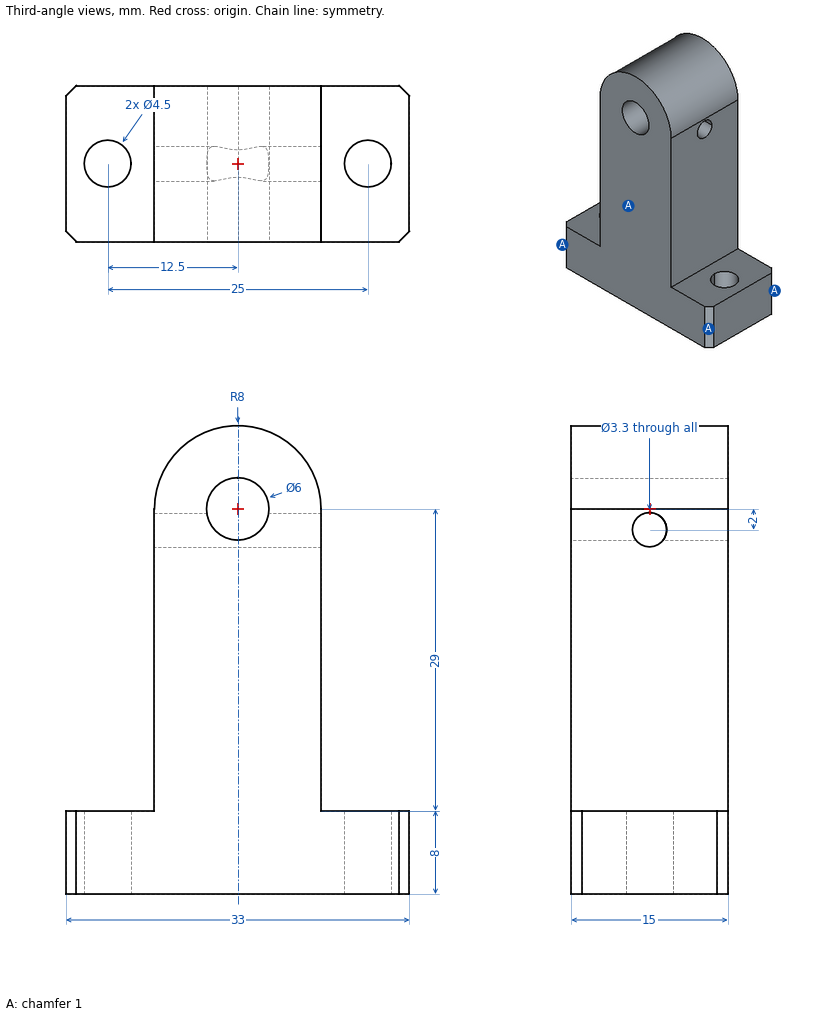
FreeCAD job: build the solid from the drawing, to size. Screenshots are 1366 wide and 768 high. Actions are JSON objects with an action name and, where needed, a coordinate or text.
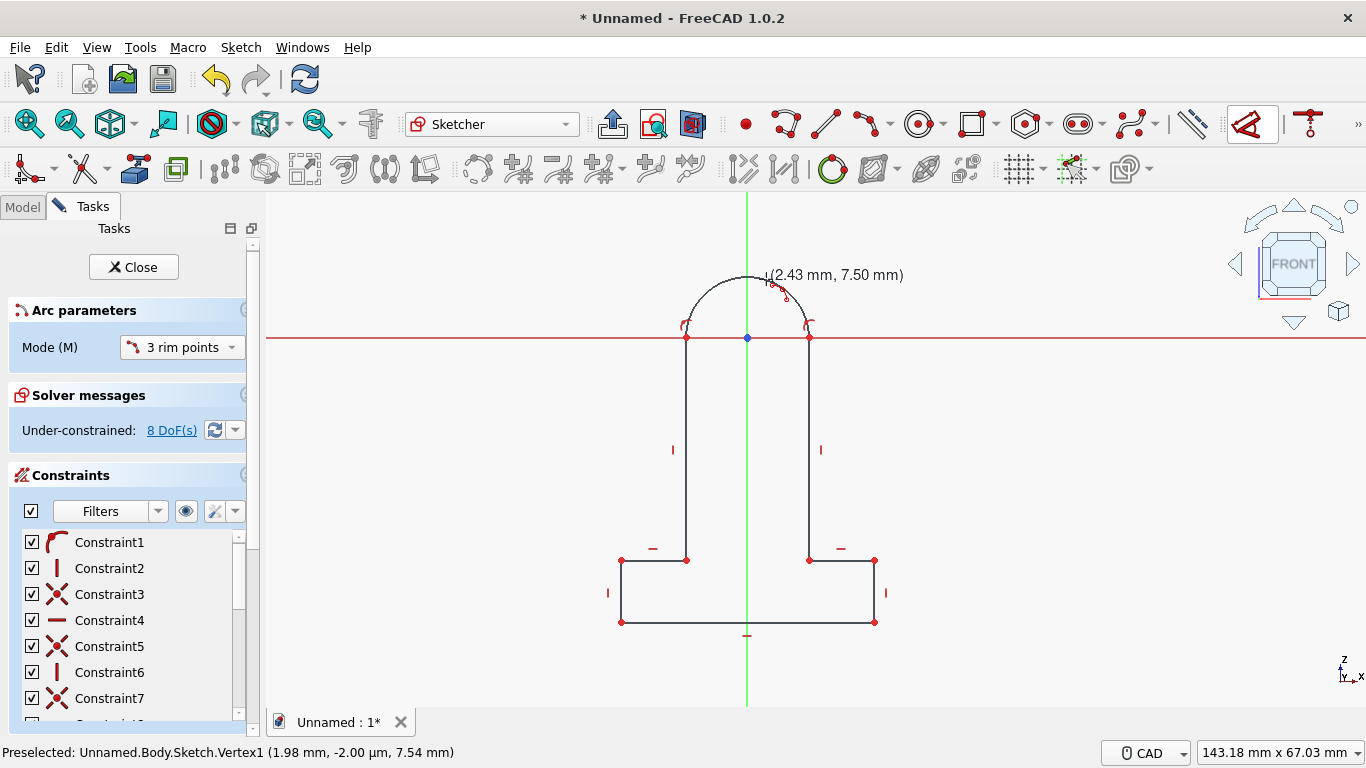
{"action": "left_click", "coordinate": [920, 124]}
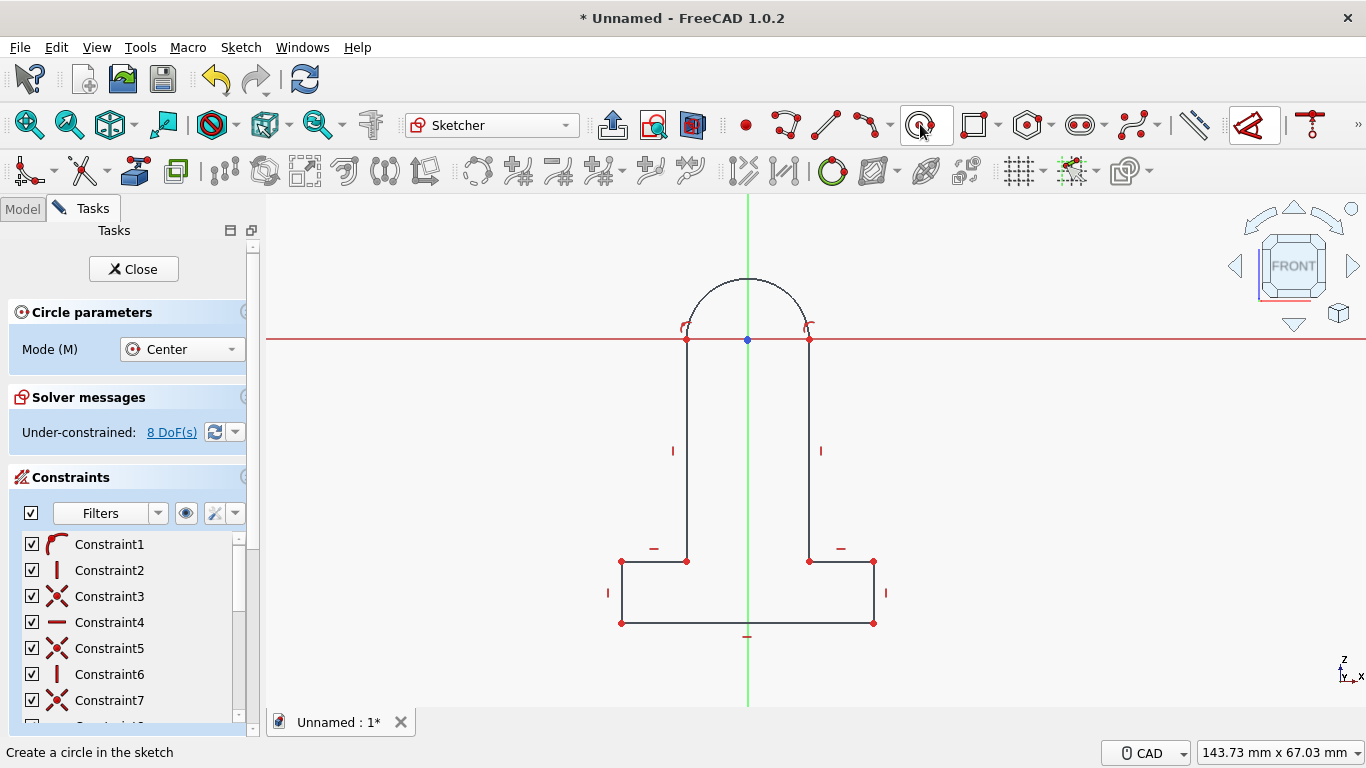
{"action": "left_click", "coordinate": [748, 339]}
{"action": "mouse_move", "coordinate": [764, 323]}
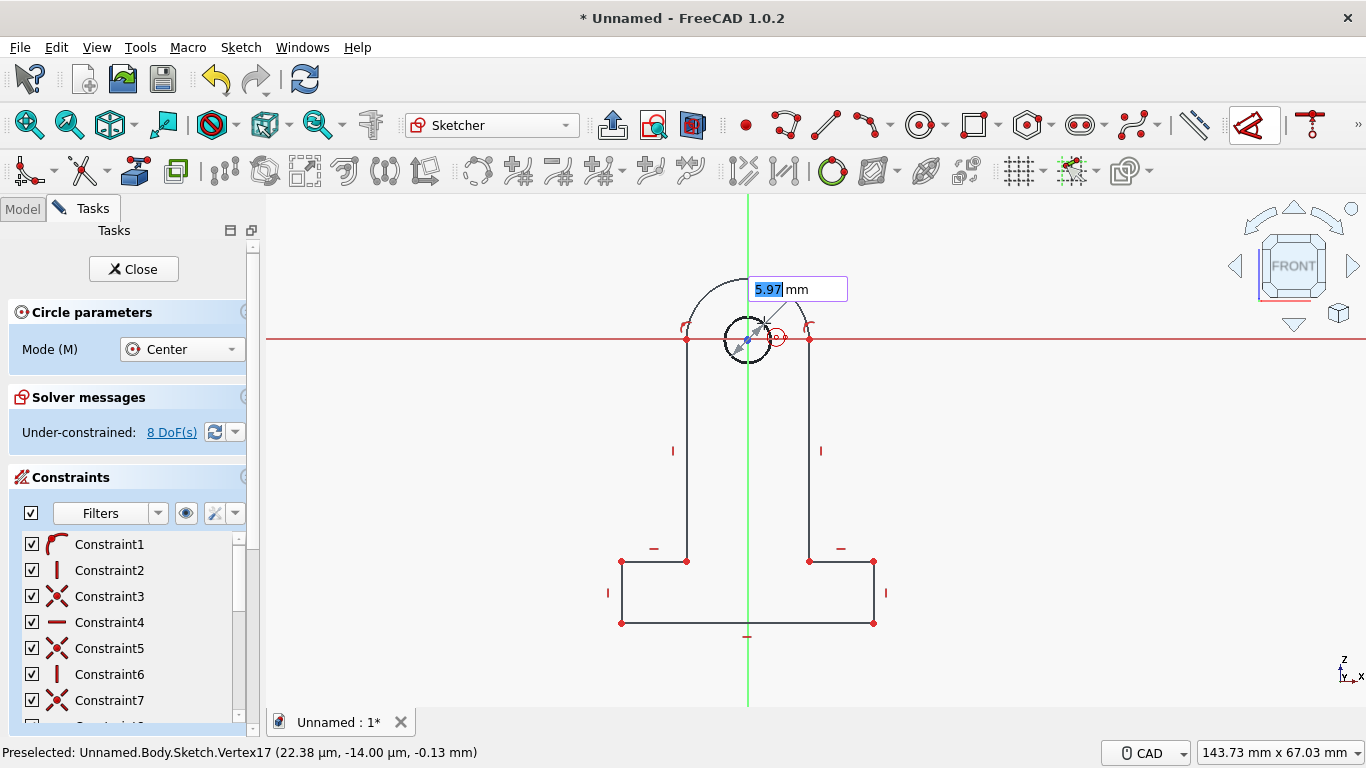
{"action": "type", "text": "6"}
{"action": "key", "text": "Return"}
{"action": "key", "text": "Escape"}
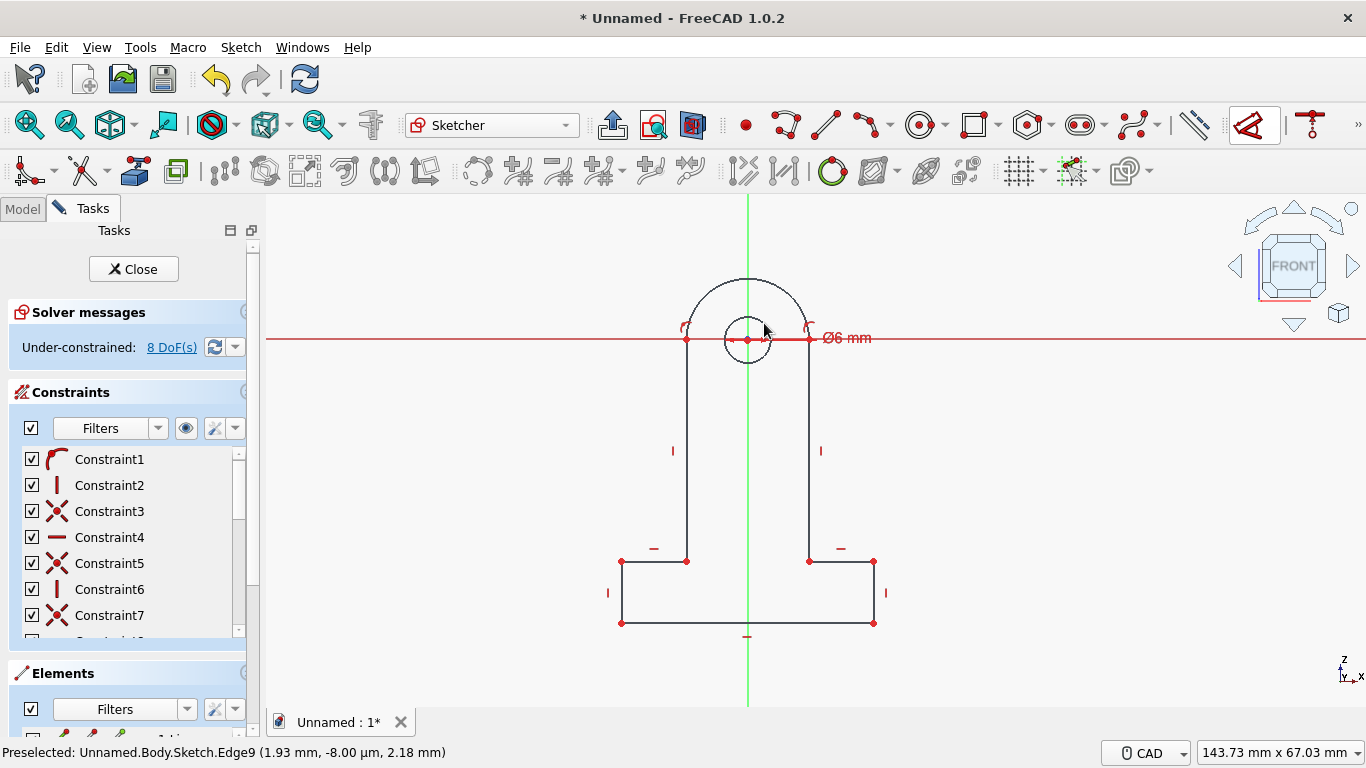
{"action": "left_click", "coordinate": [809, 406]}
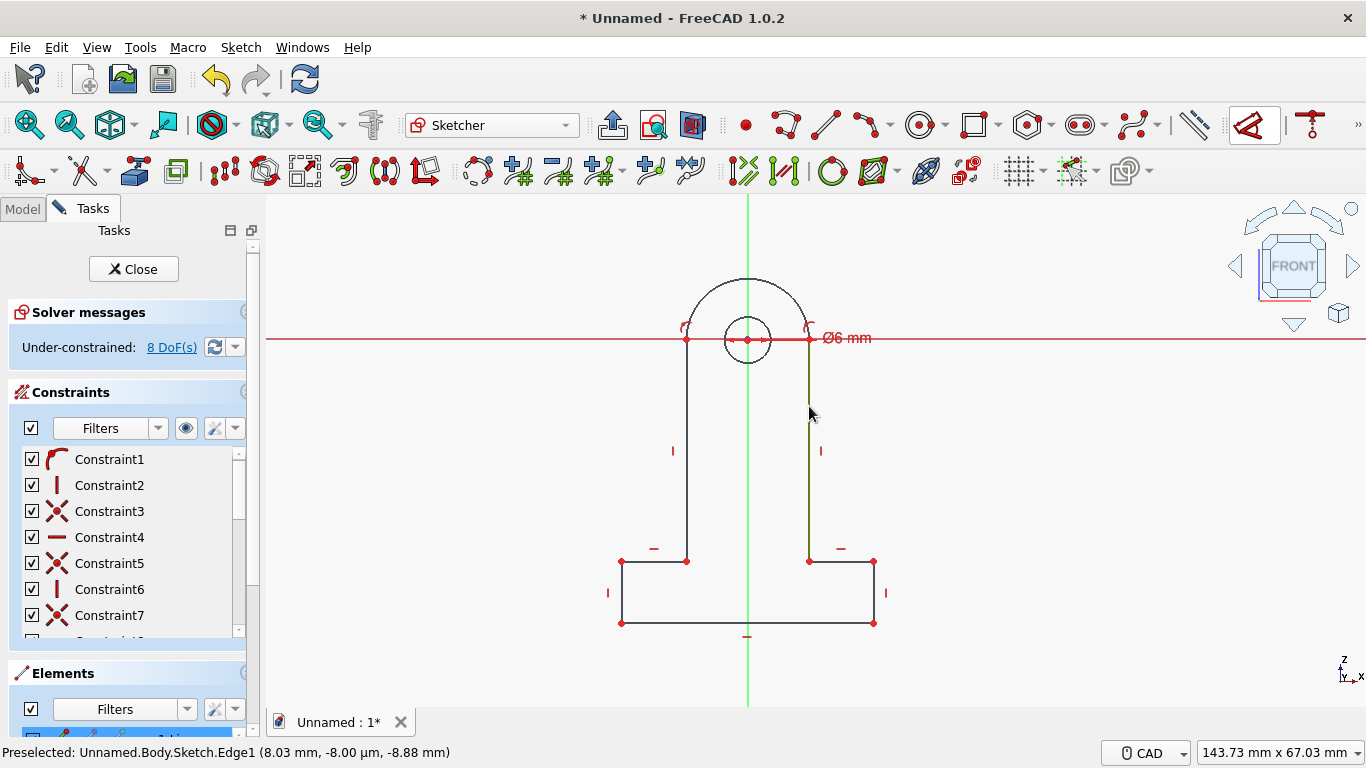
{"action": "left_click", "coordinate": [783, 290]}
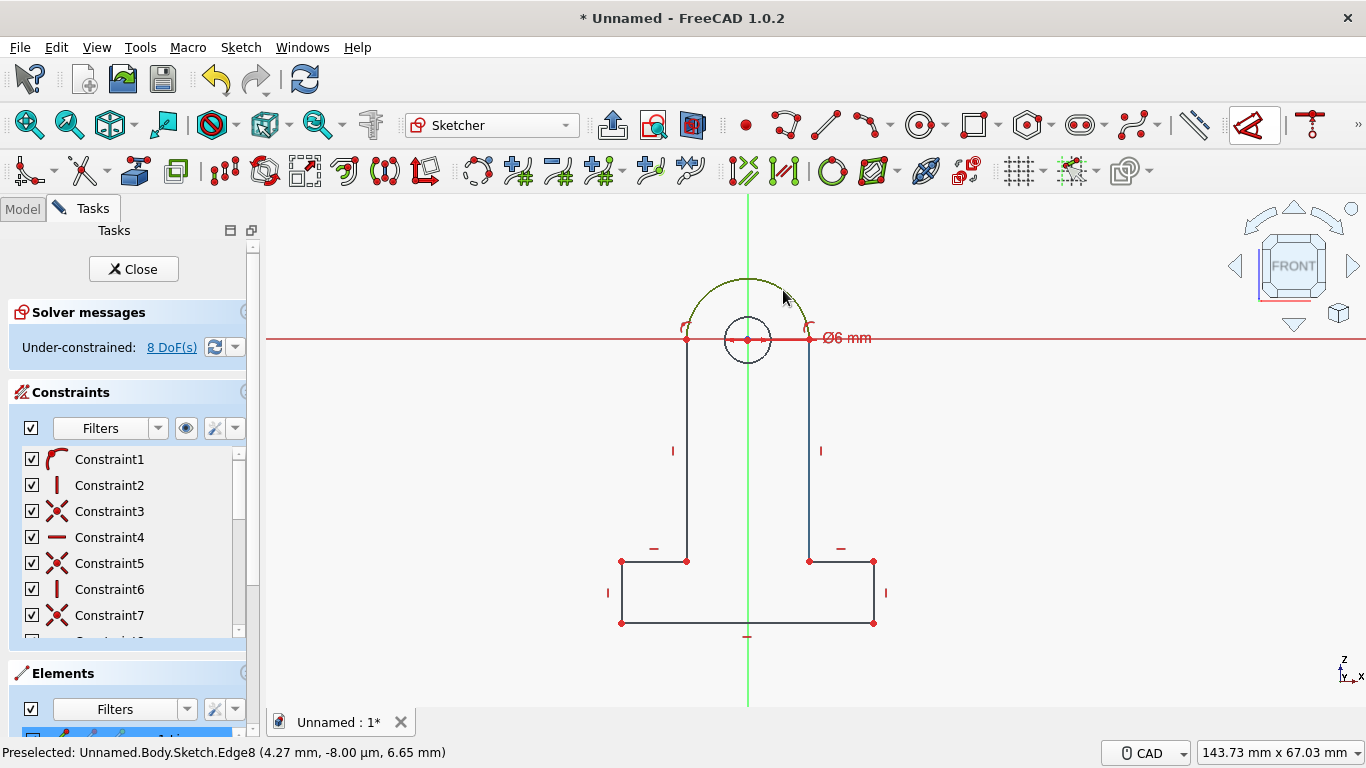
{"action": "key", "text": "t"}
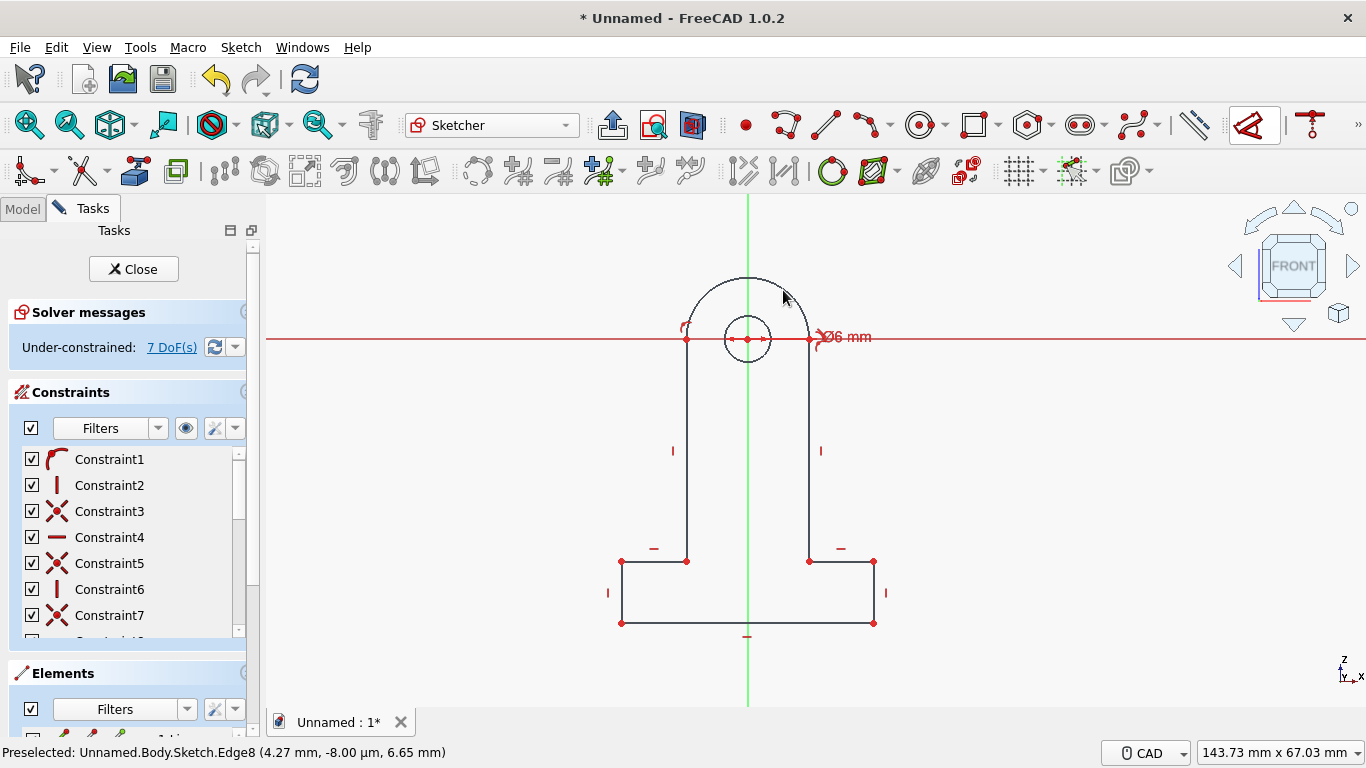
{"action": "left_click", "coordinate": [748, 339]}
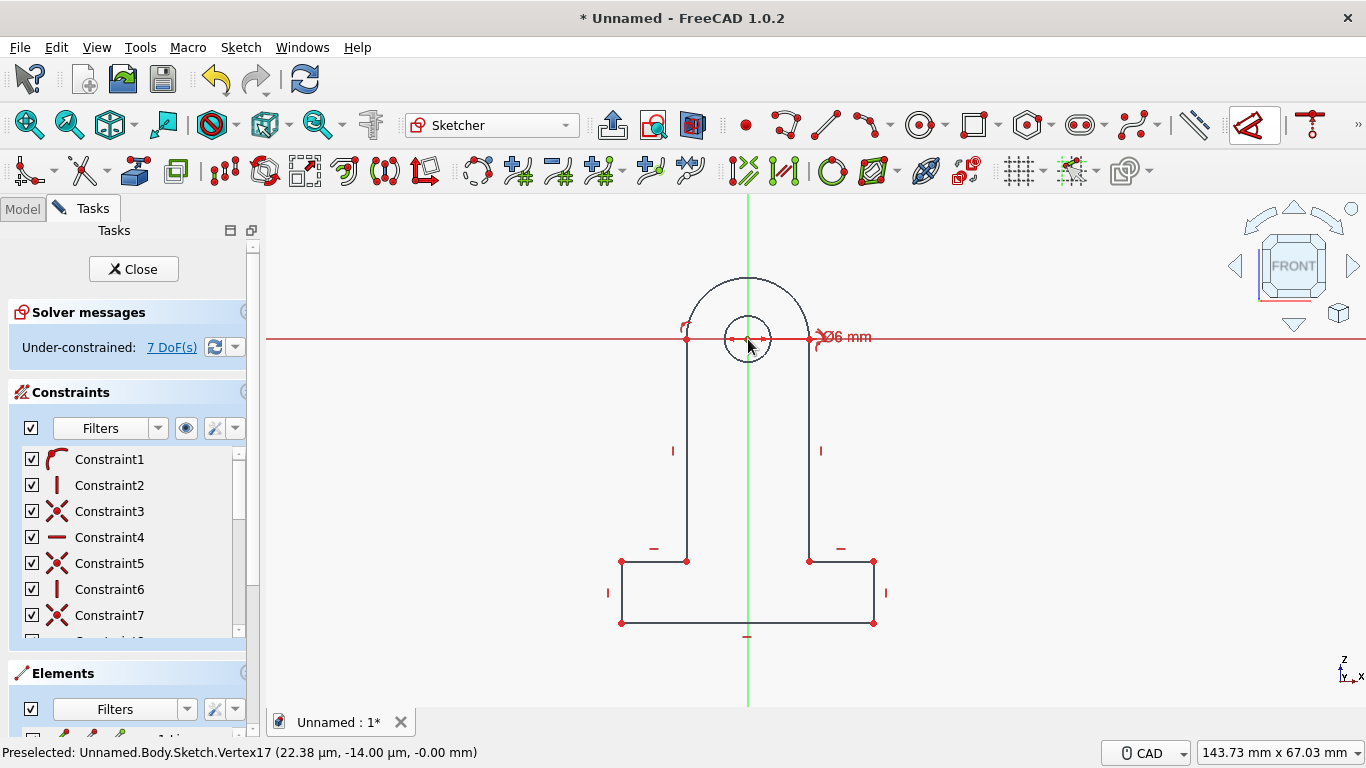
{"action": "left_click", "coordinate": [748, 581]}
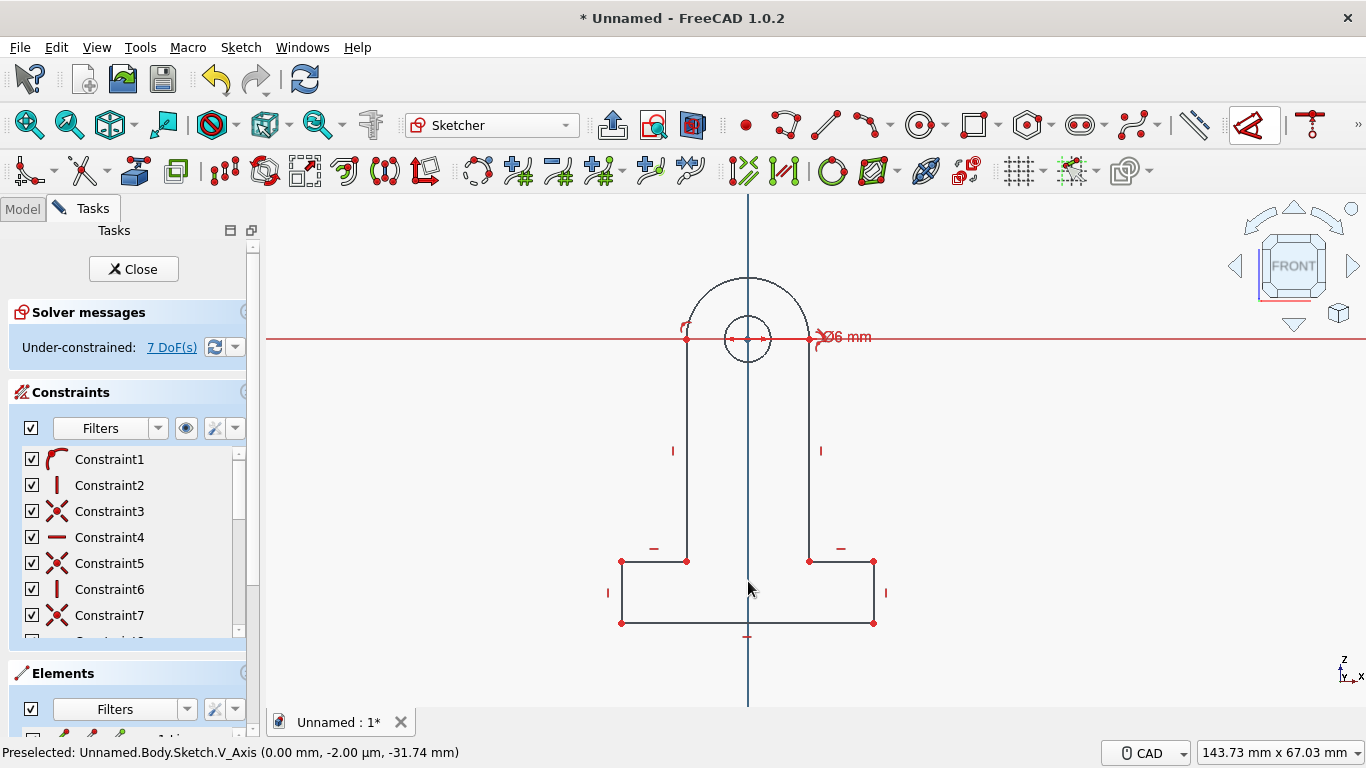
{"action": "key", "text": "c"}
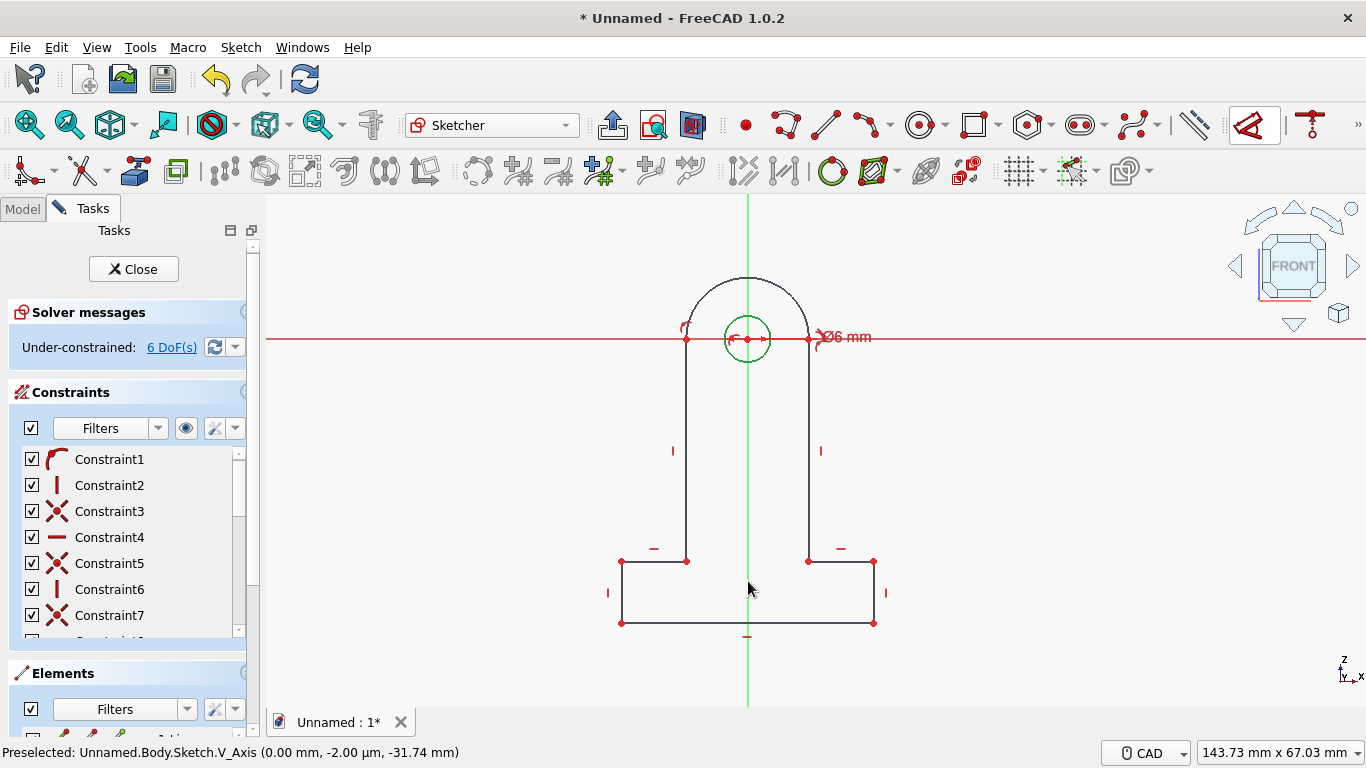
{"action": "left_click", "coordinate": [874, 562]}